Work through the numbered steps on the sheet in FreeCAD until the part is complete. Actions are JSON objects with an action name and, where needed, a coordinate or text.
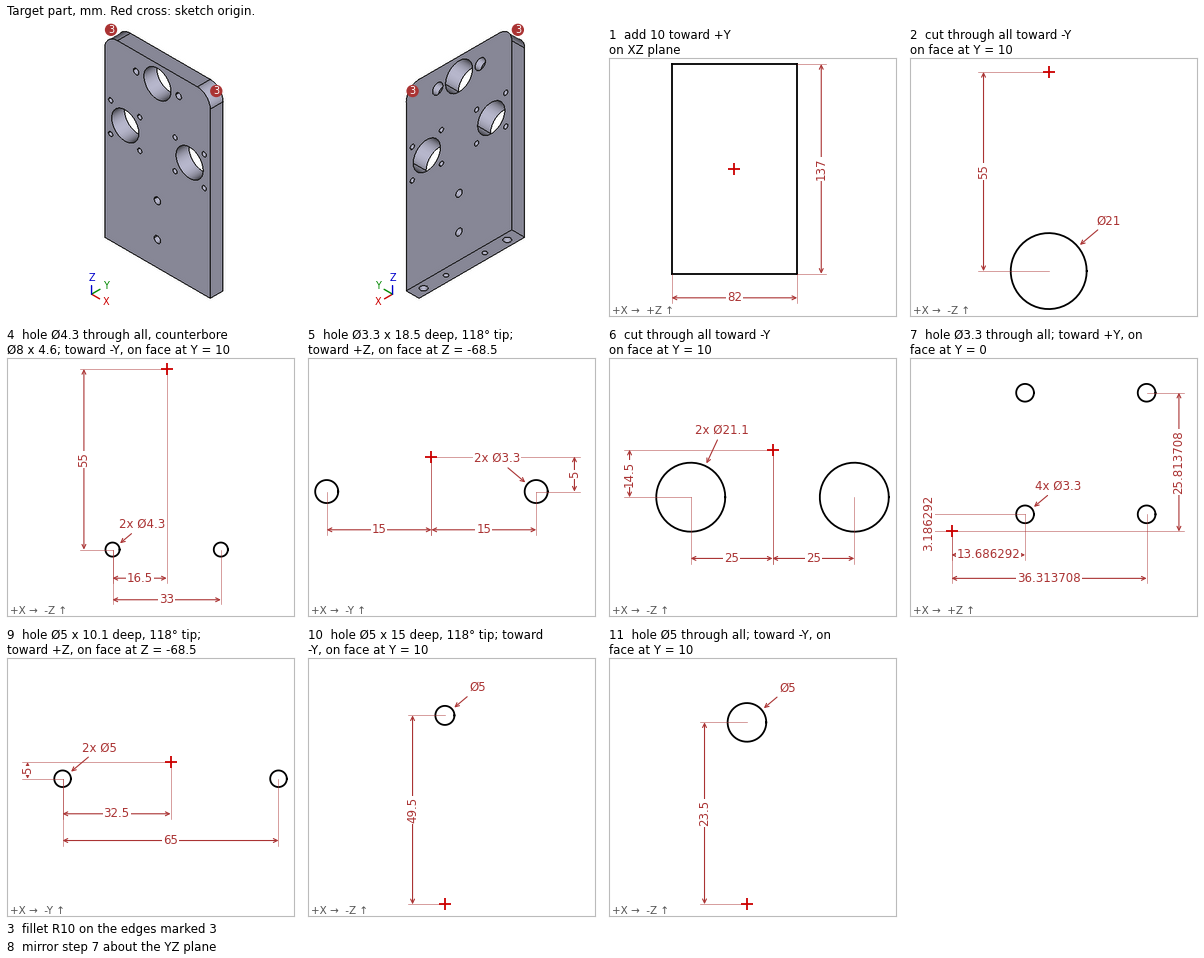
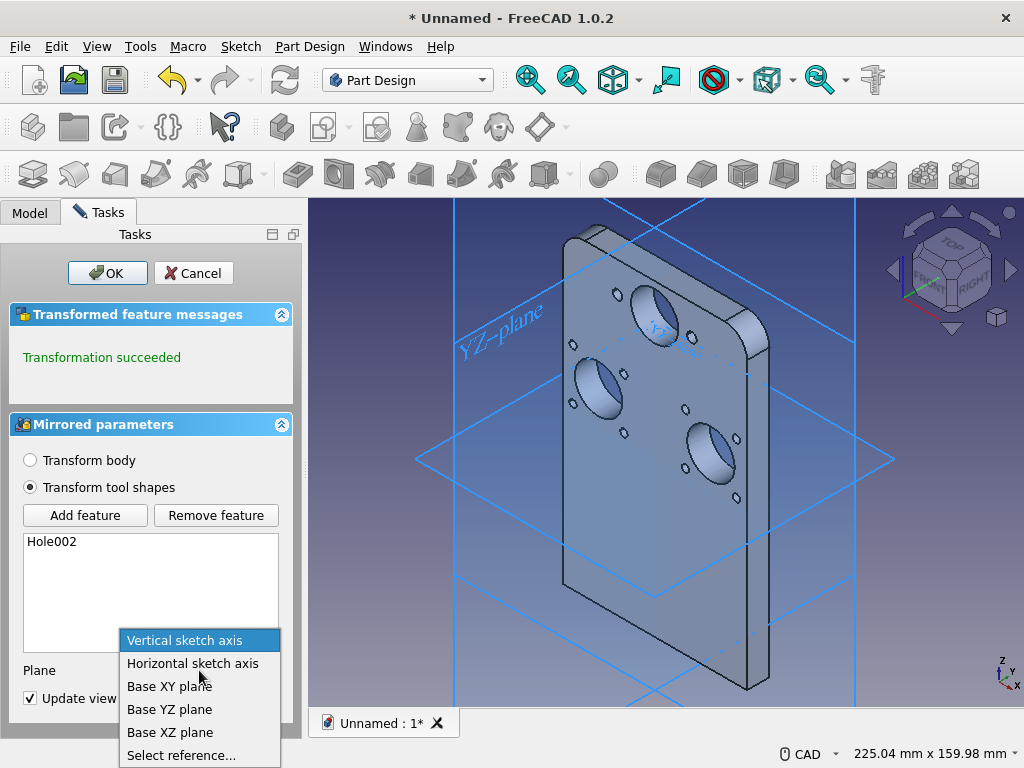
{"action": "left_click", "coordinate": [198, 710]}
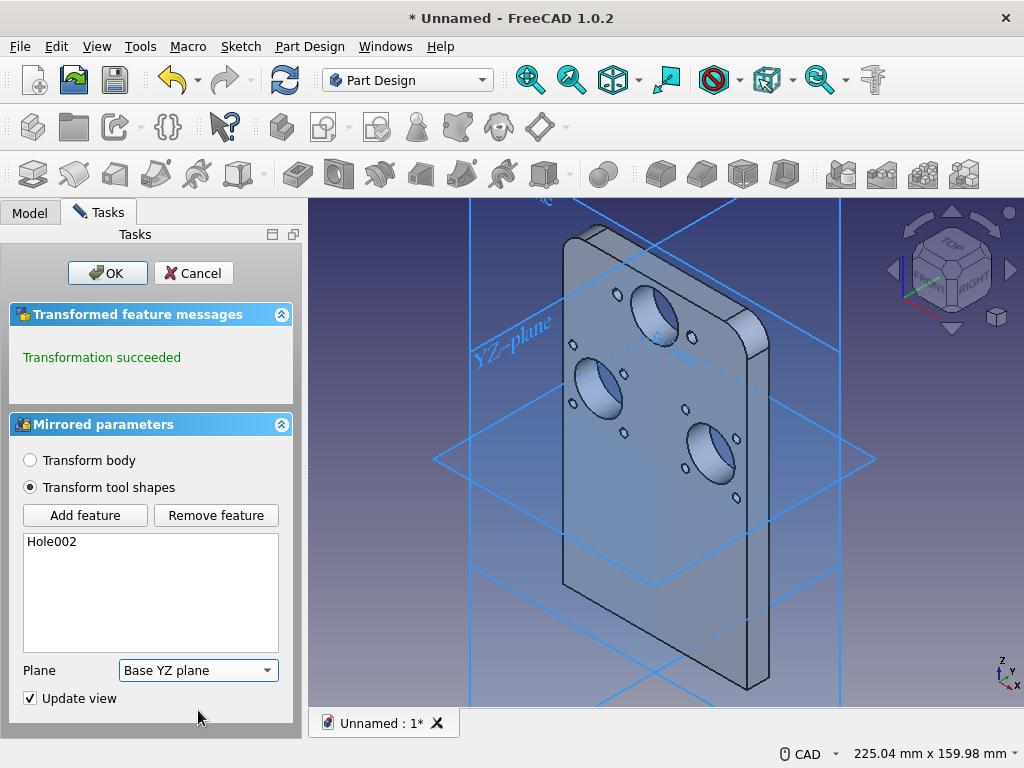
{"action": "left_click", "coordinate": [108, 273]}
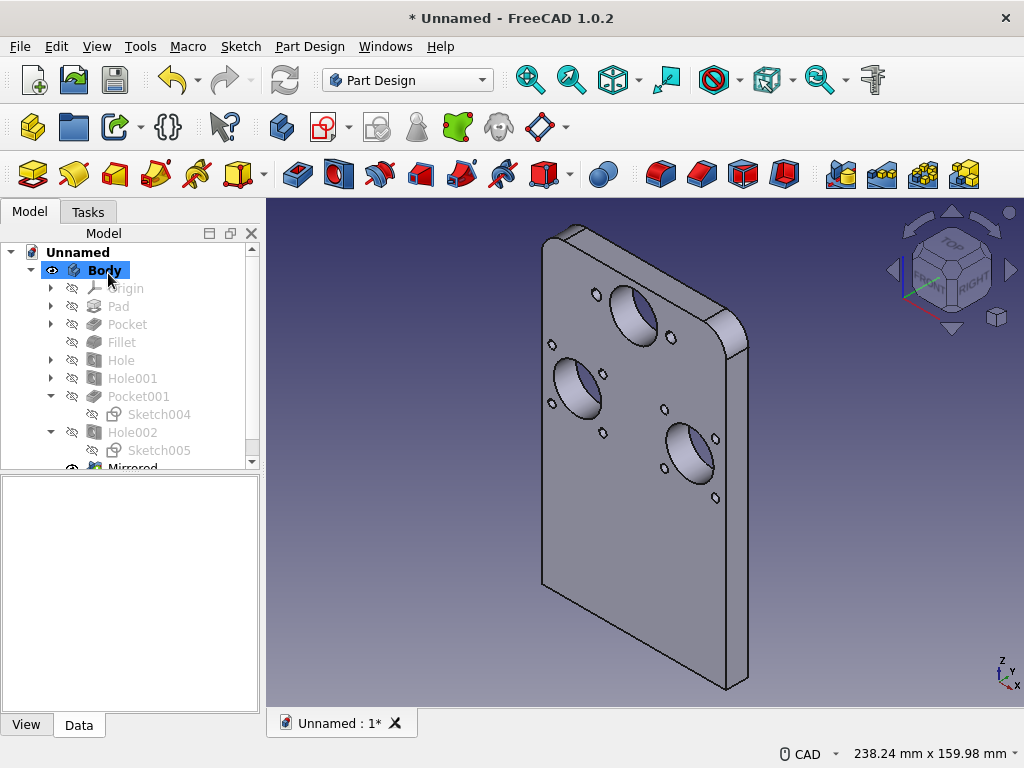
{"action": "key", "text": "5"}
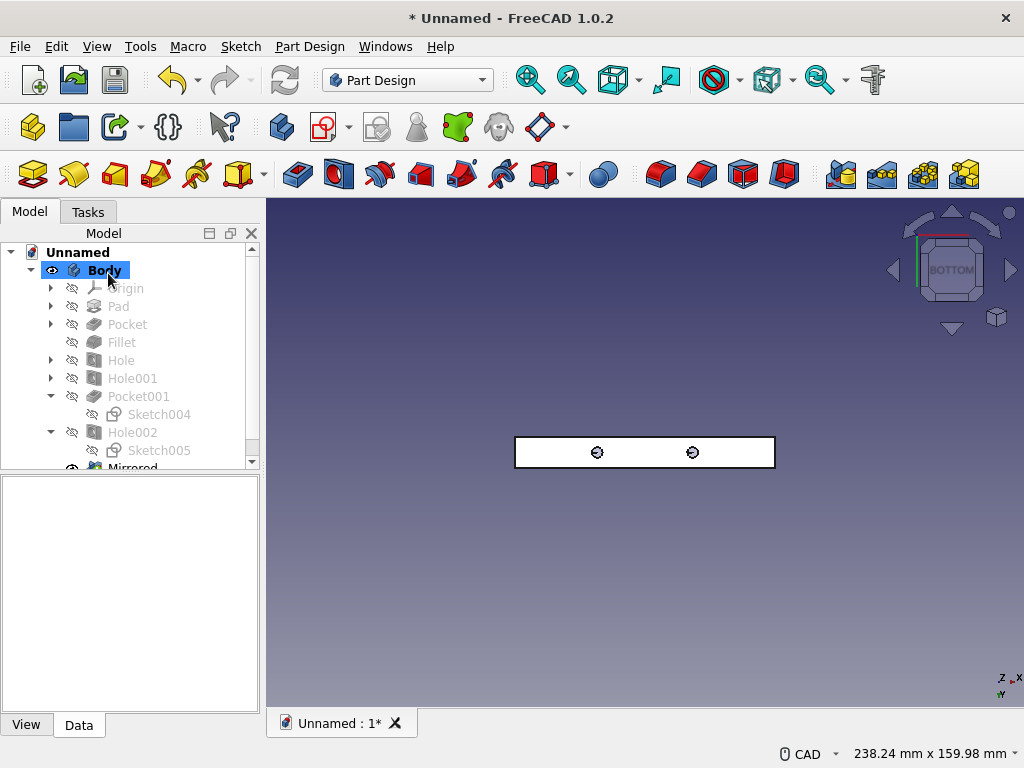
{"action": "key", "text": "v f"}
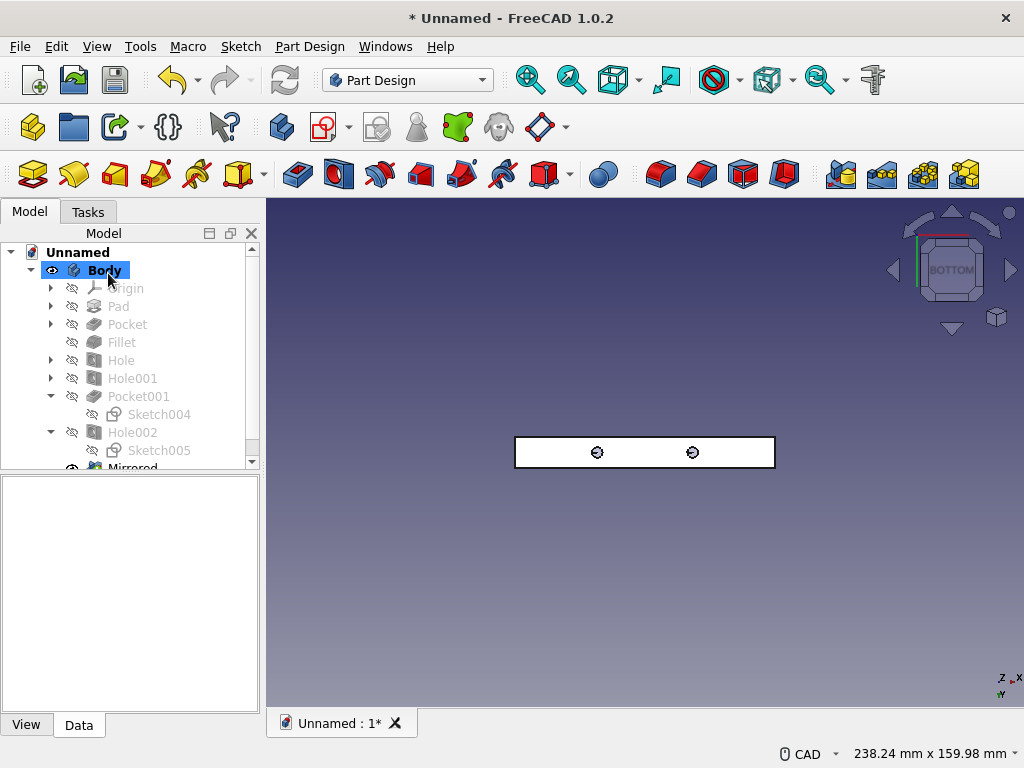
{"action": "left_click", "coordinate": [757, 451]}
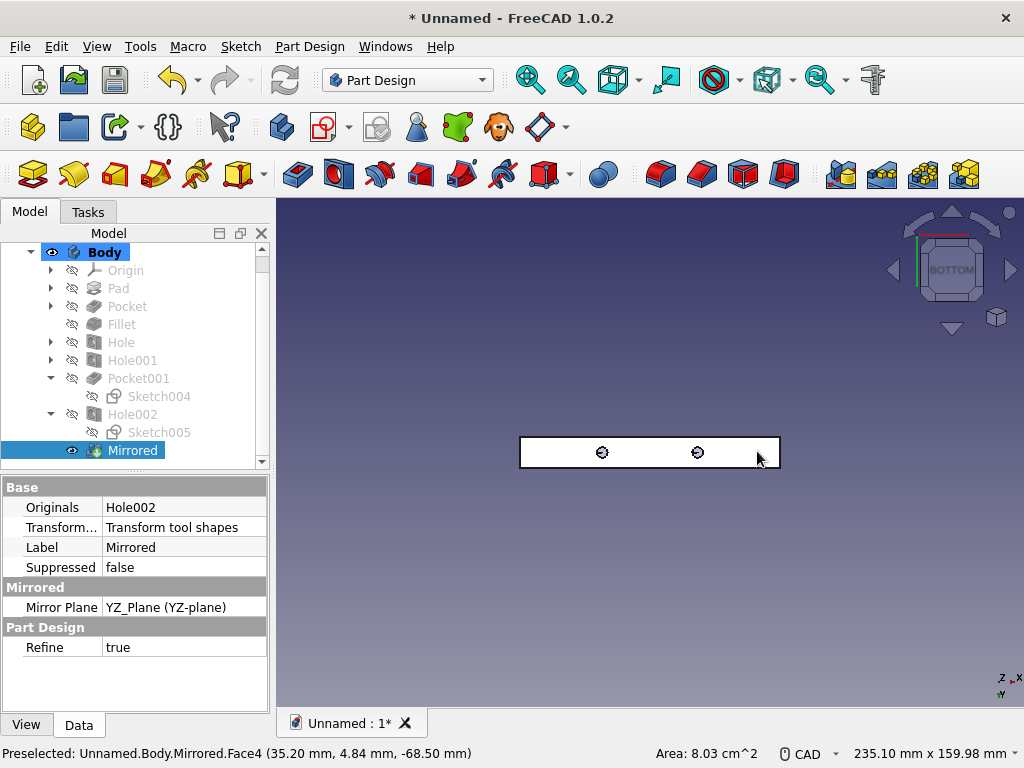
{"action": "left_click", "coordinate": [322, 128]}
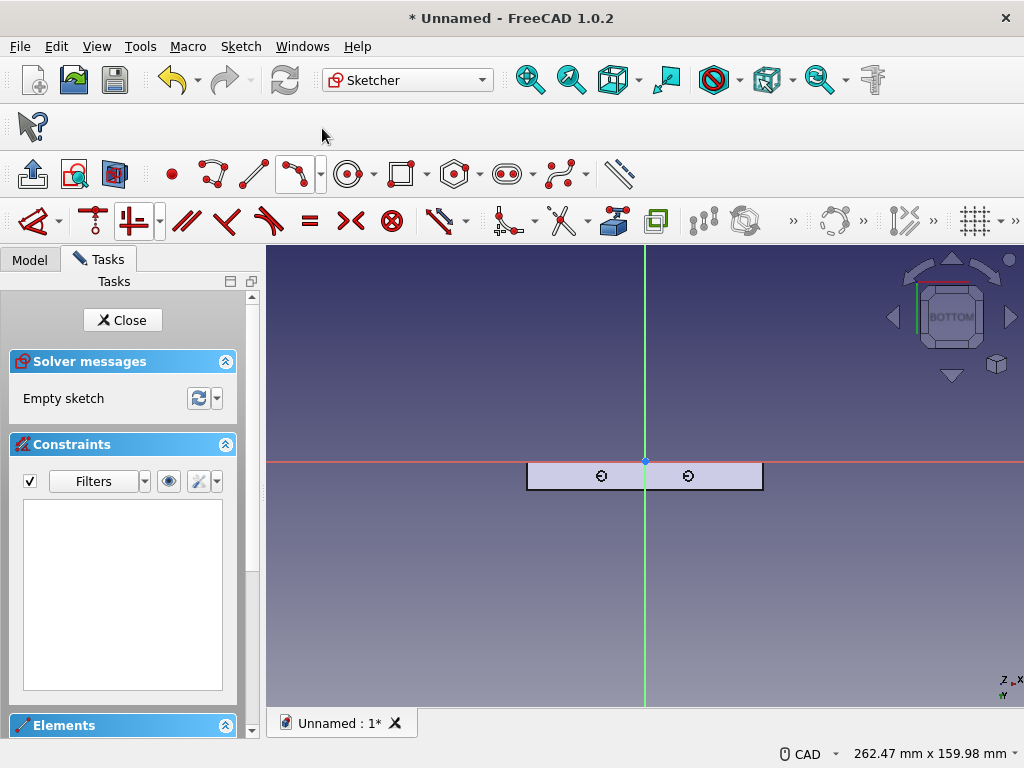
{"action": "scroll", "coordinate": [728, 468], "scroll_direction": "up", "scroll_amount": 3}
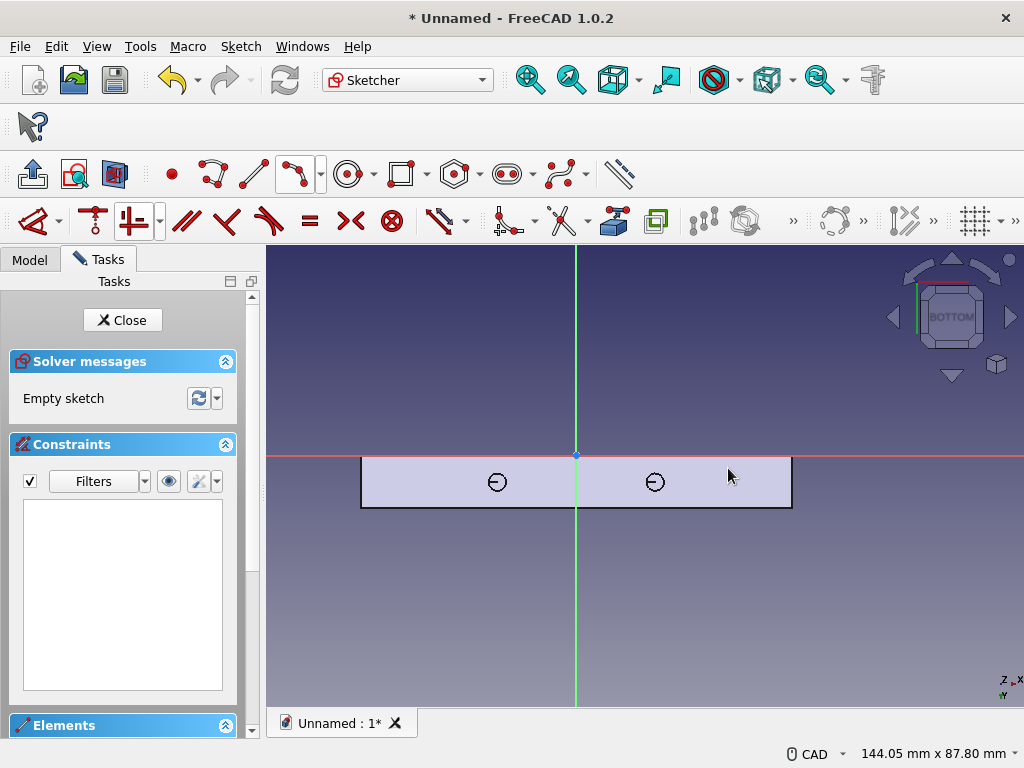
{"action": "key", "text": "g c"}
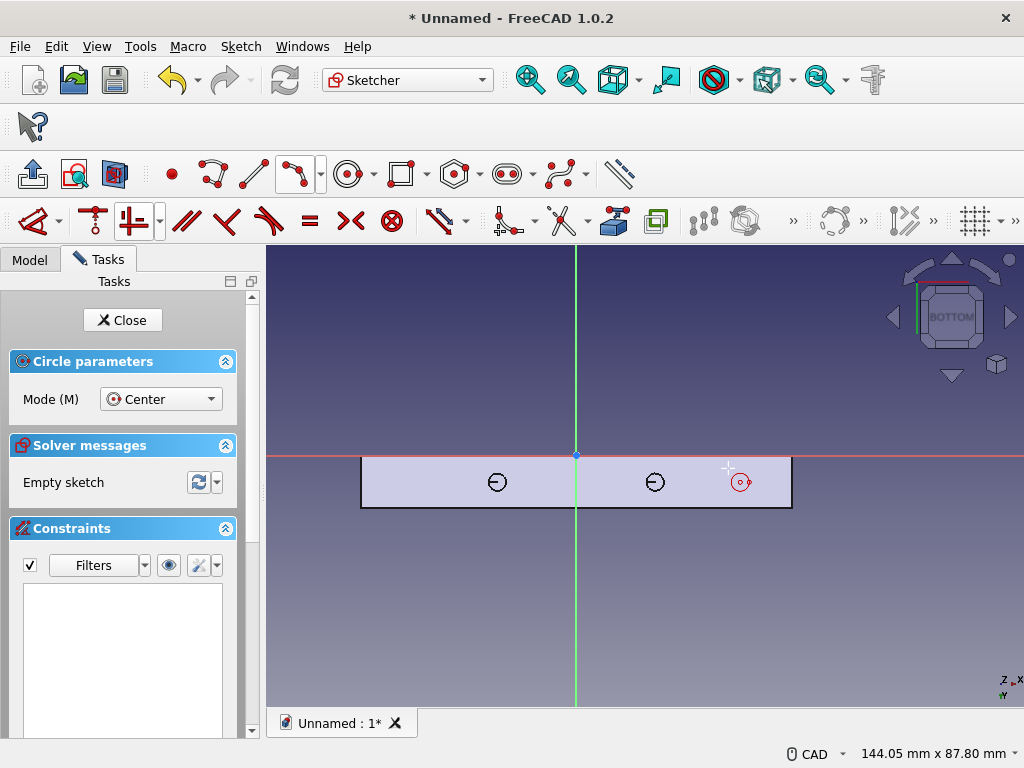
{"action": "scroll", "coordinate": [405, 482], "scroll_direction": "up", "scroll_amount": 3}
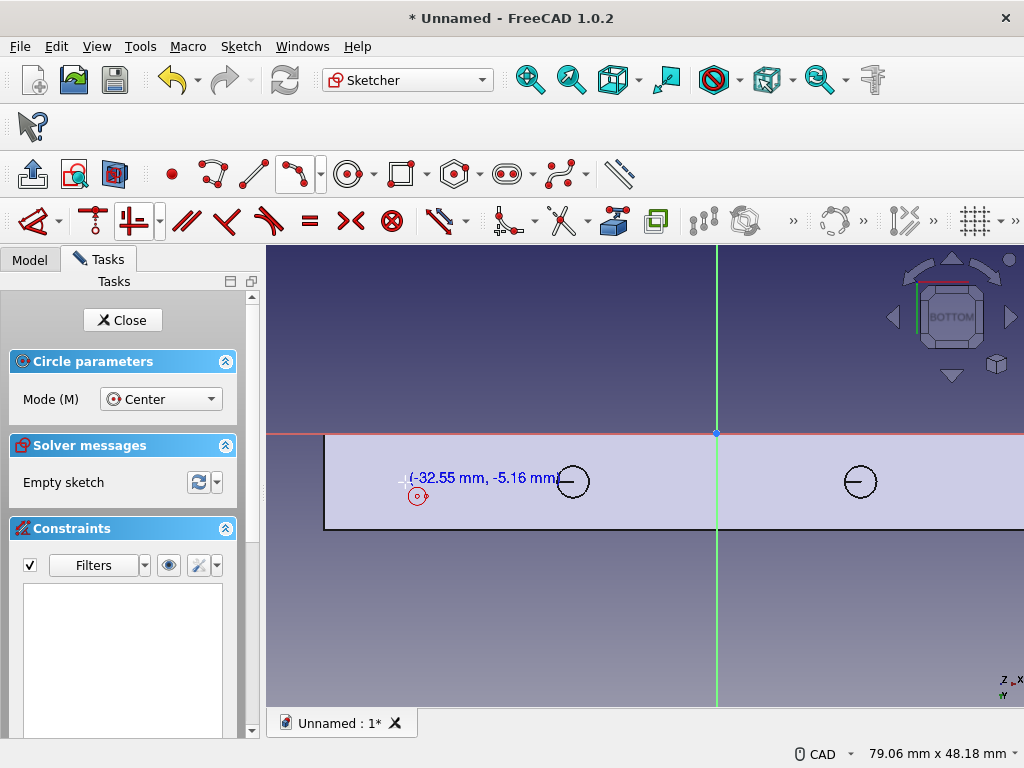
{"action": "left_click", "coordinate": [405, 482]}
{"action": "mouse_move", "coordinate": [422, 465]}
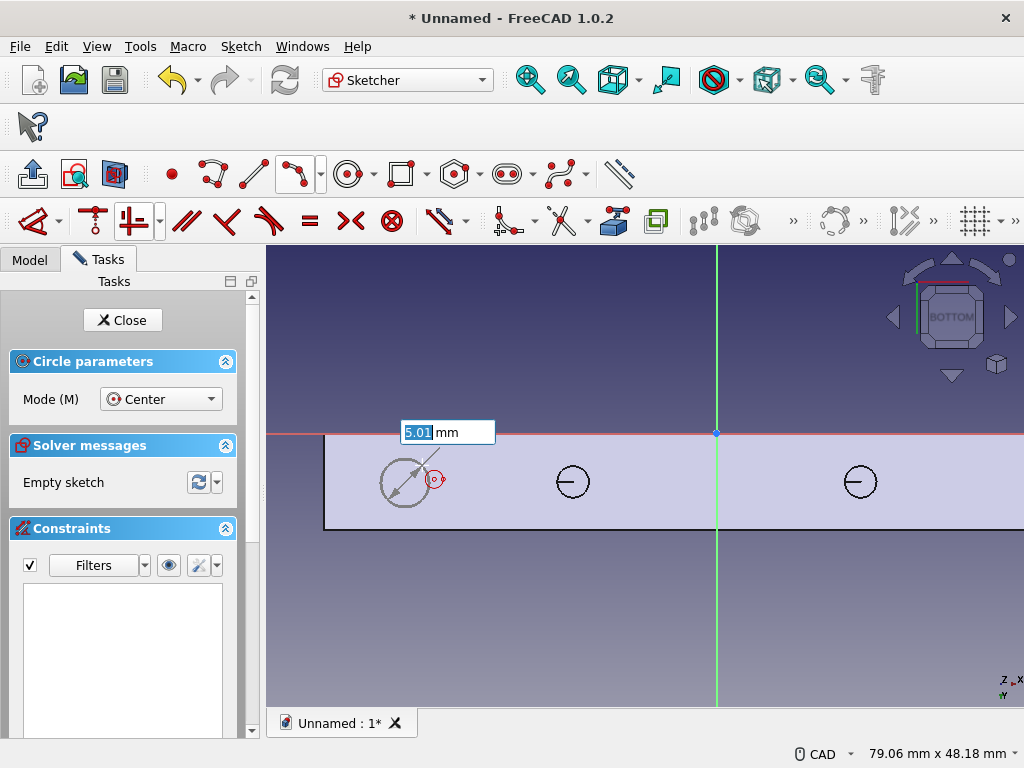
{"action": "type", "text": "5"}
{"action": "key", "text": "Return"}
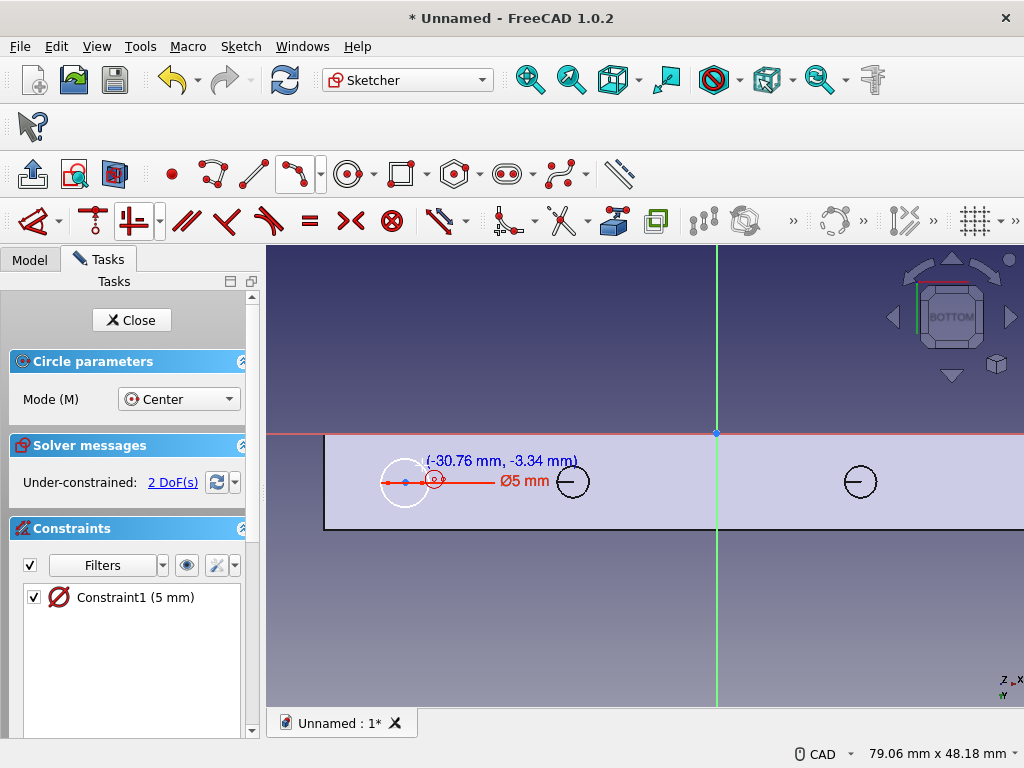
{"action": "scroll", "coordinate": [406, 483], "scroll_direction": "down", "scroll_amount": 3}